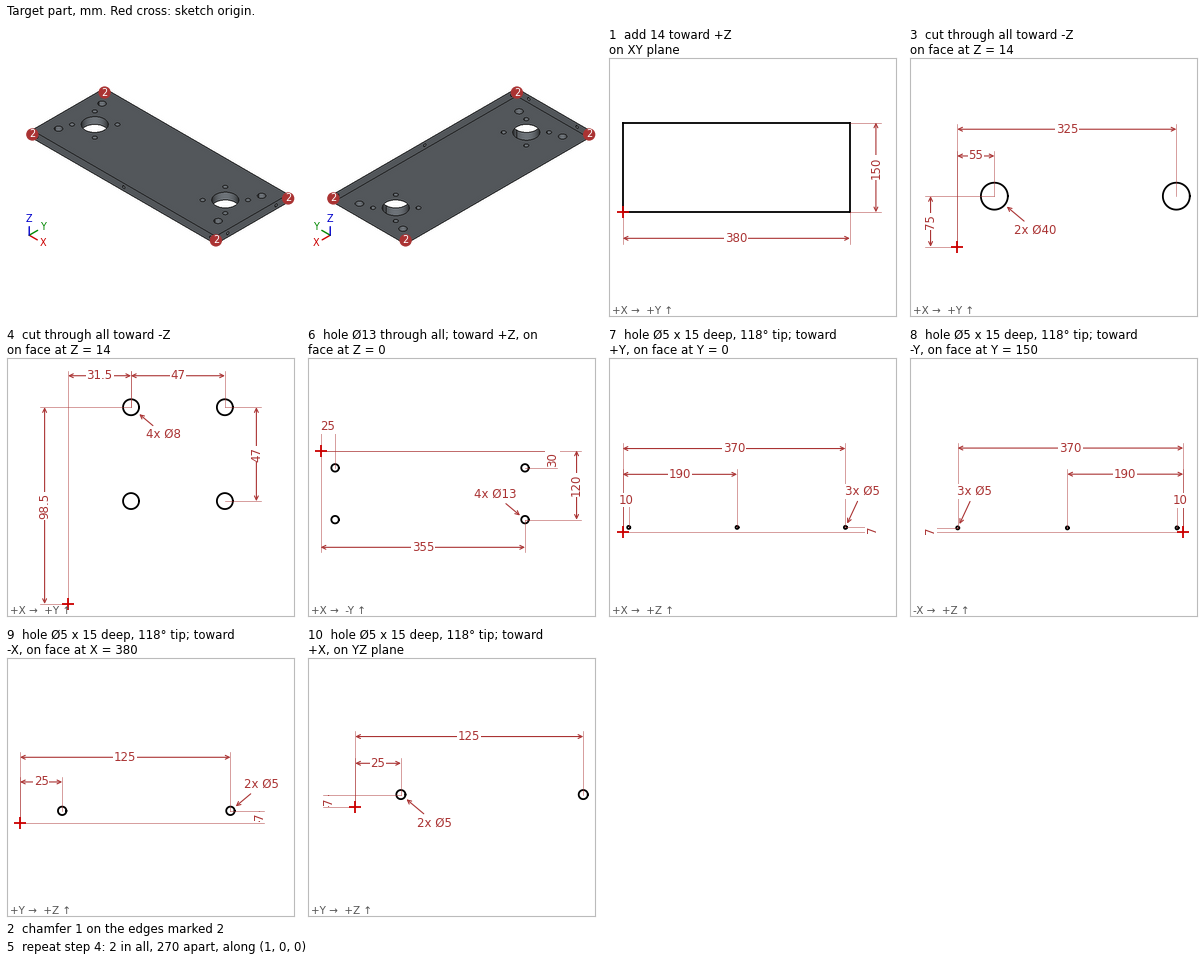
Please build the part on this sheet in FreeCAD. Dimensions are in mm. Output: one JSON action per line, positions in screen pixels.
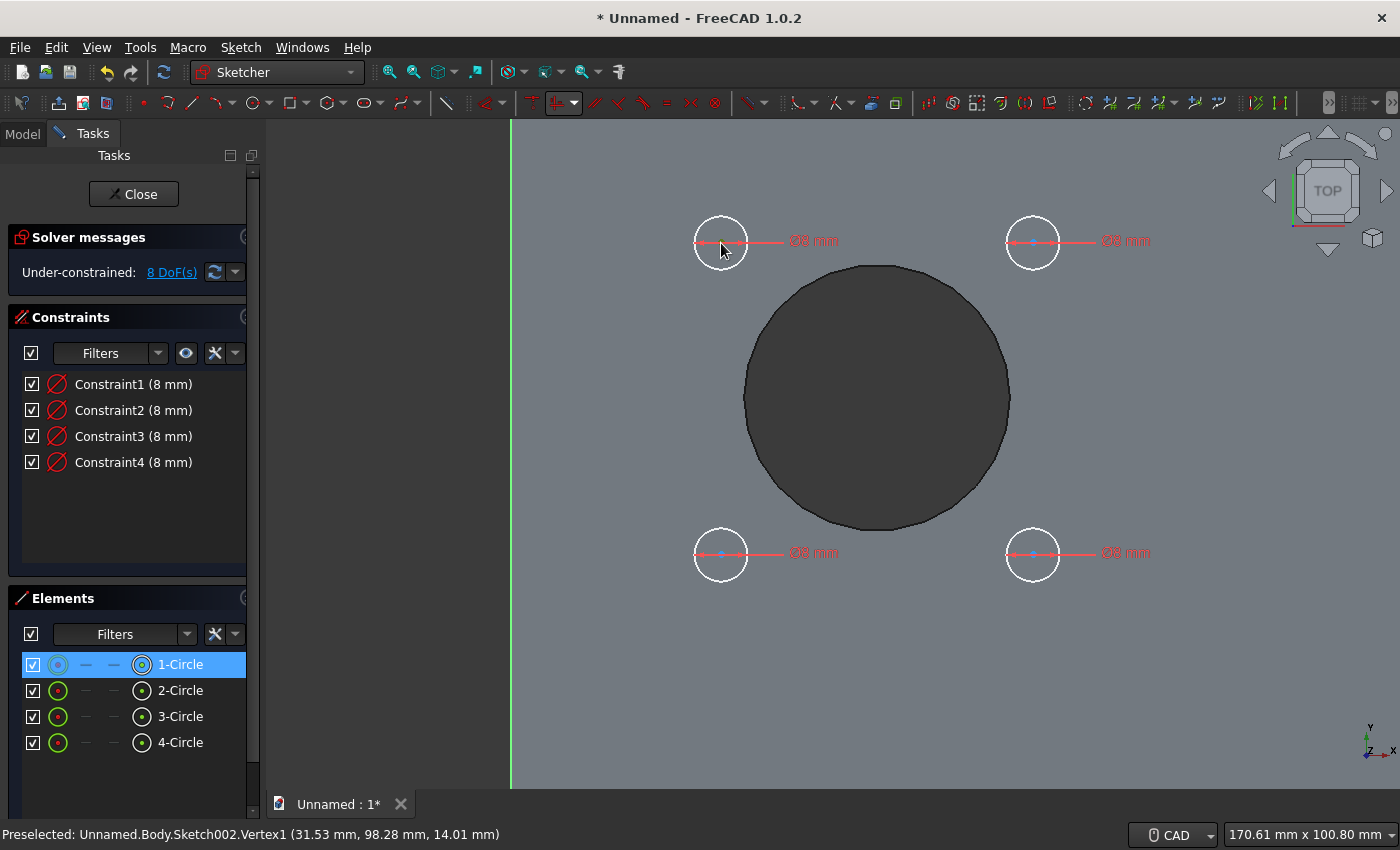
{"action": "left_click", "coordinate": [1033, 243]}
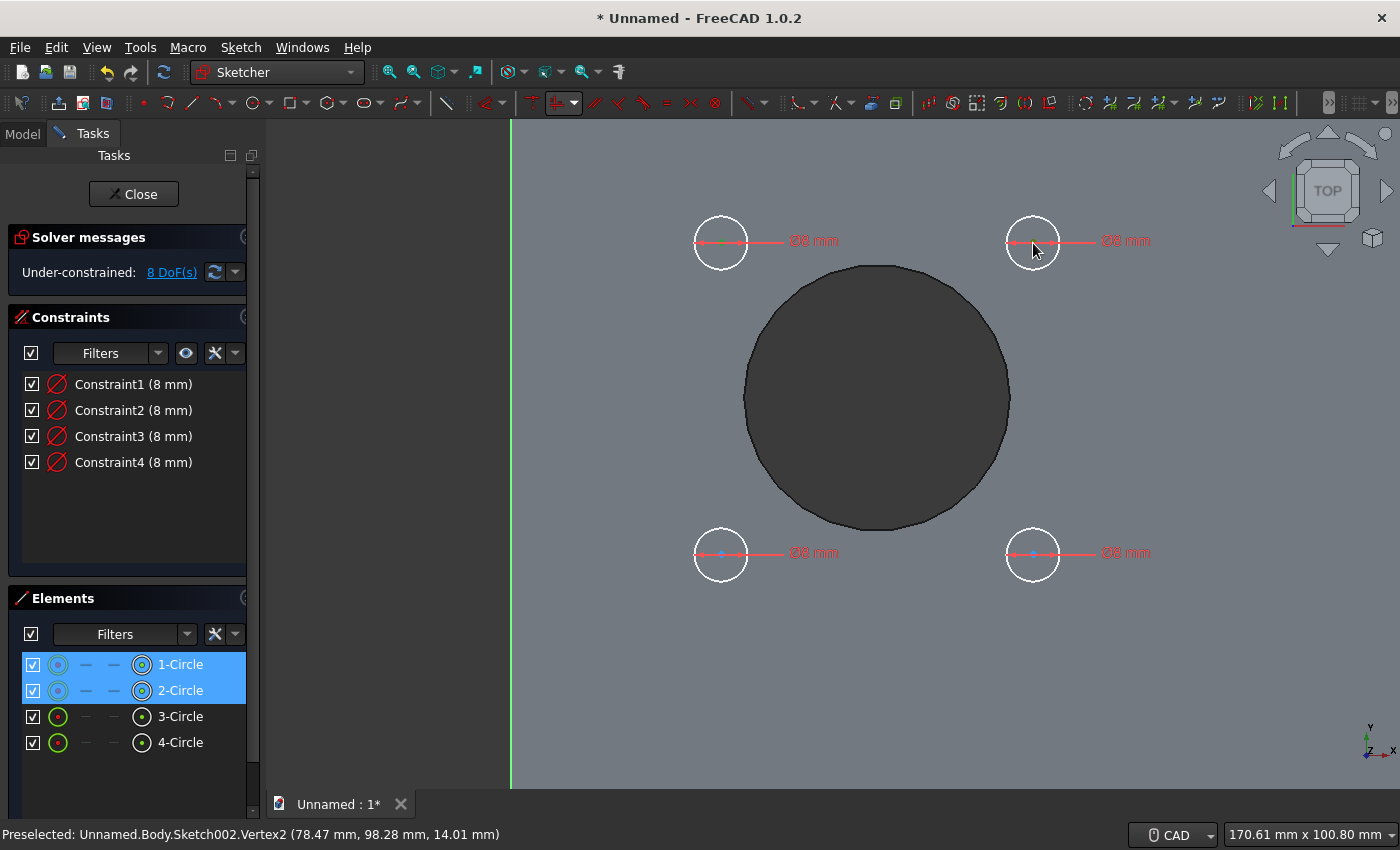
{"action": "left_click", "coordinate": [576, 104]}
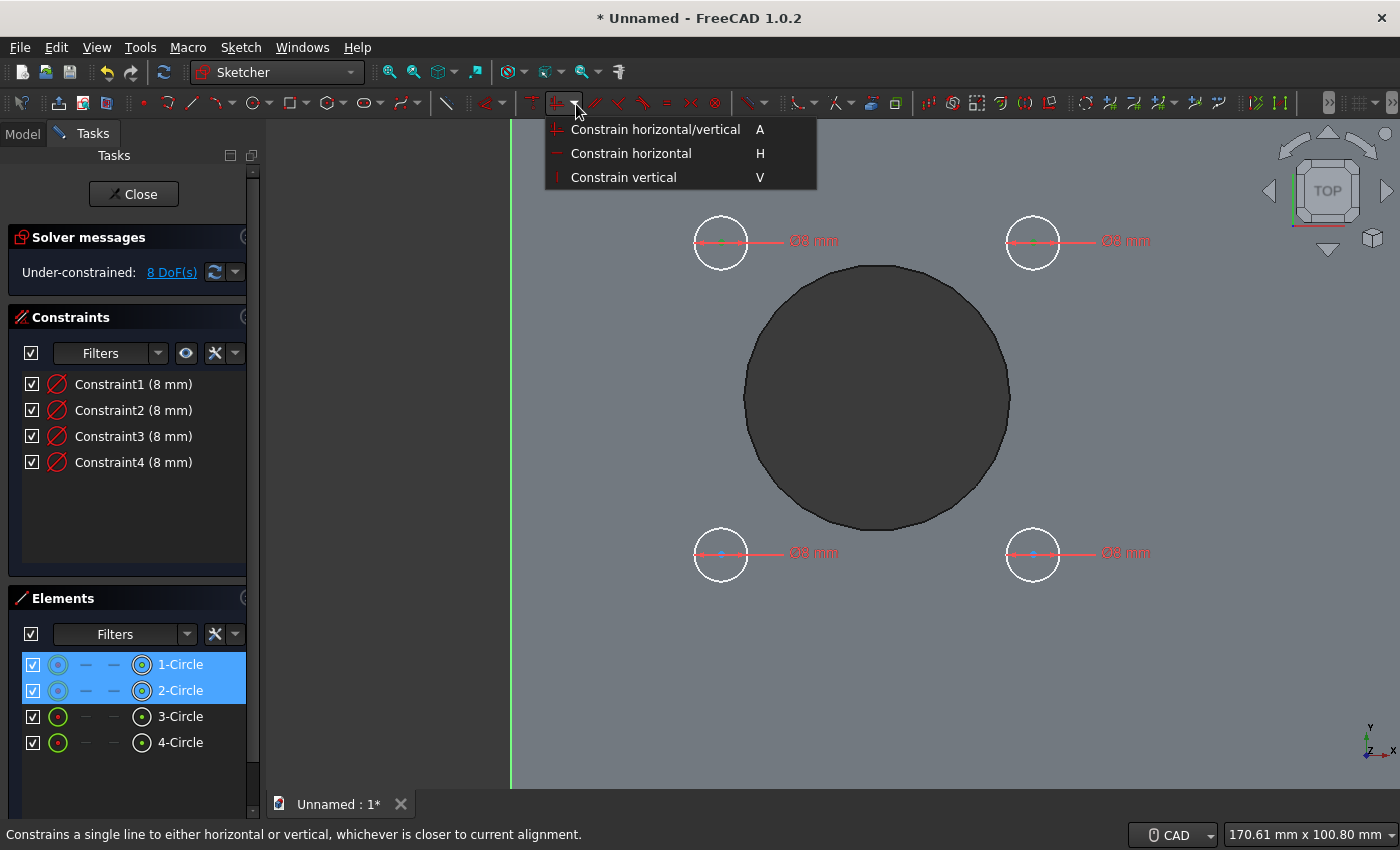
{"action": "left_click", "coordinate": [681, 153]}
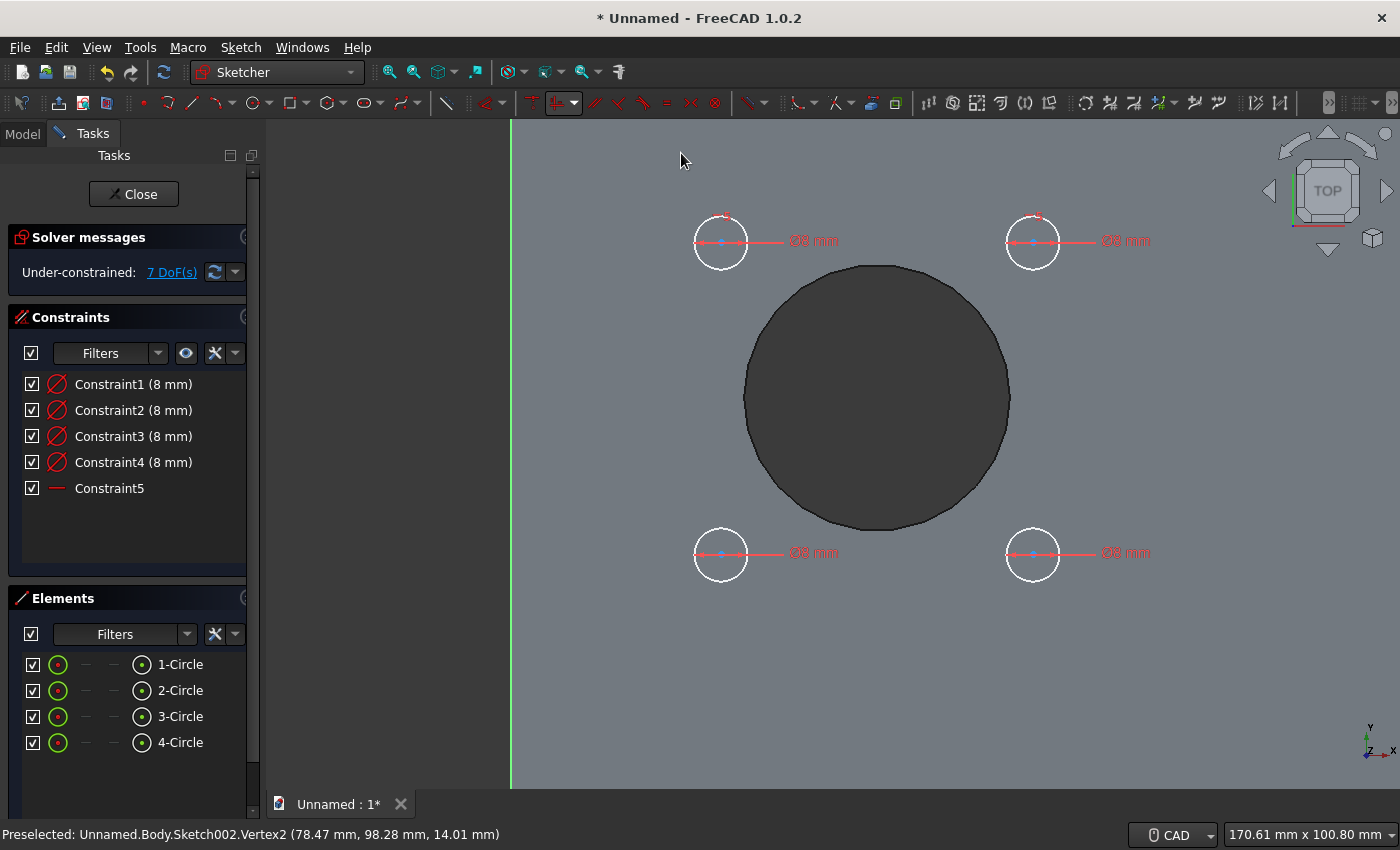
{"action": "left_click", "coordinate": [1033, 243]}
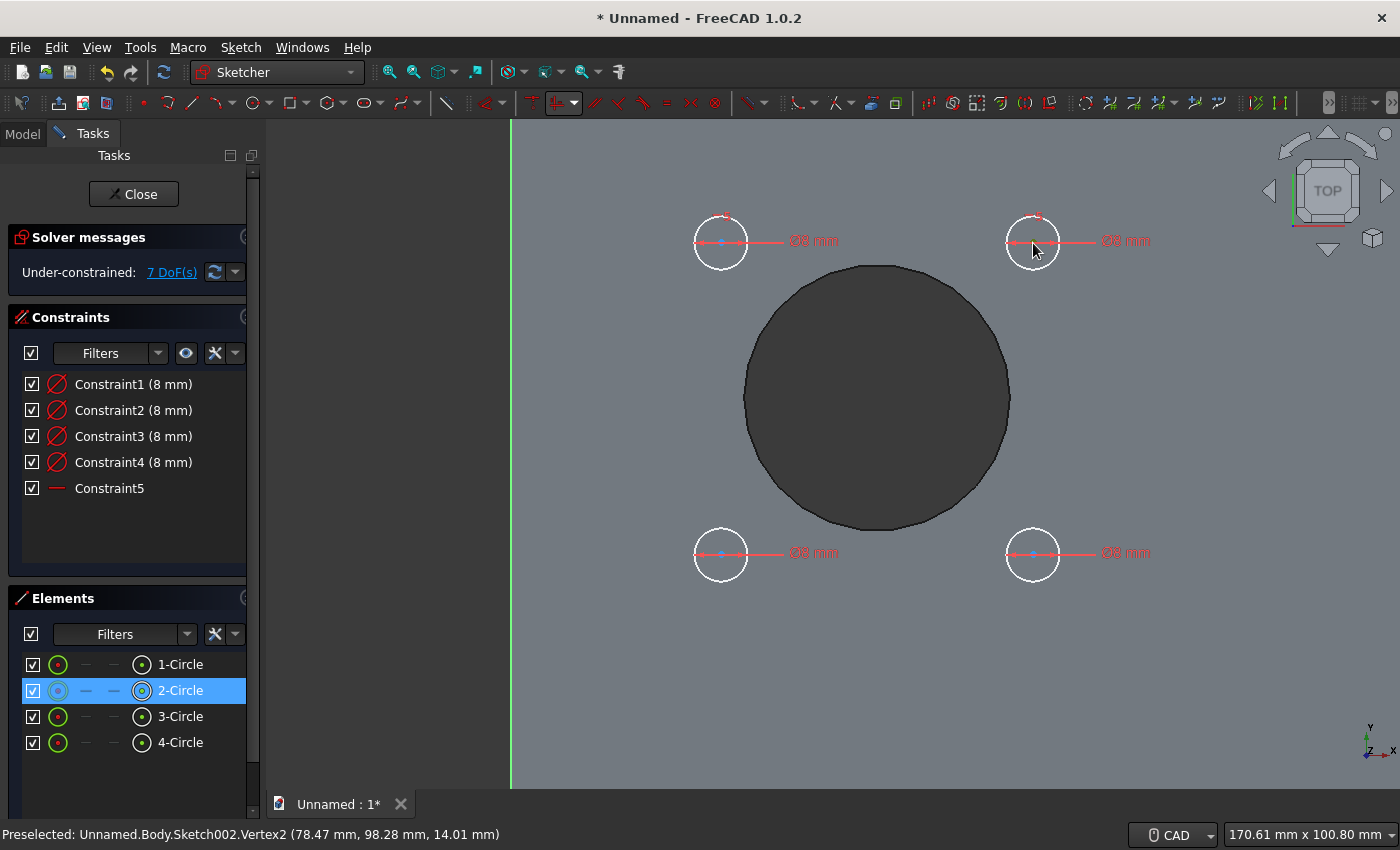
{"action": "left_click", "coordinate": [1033, 555]}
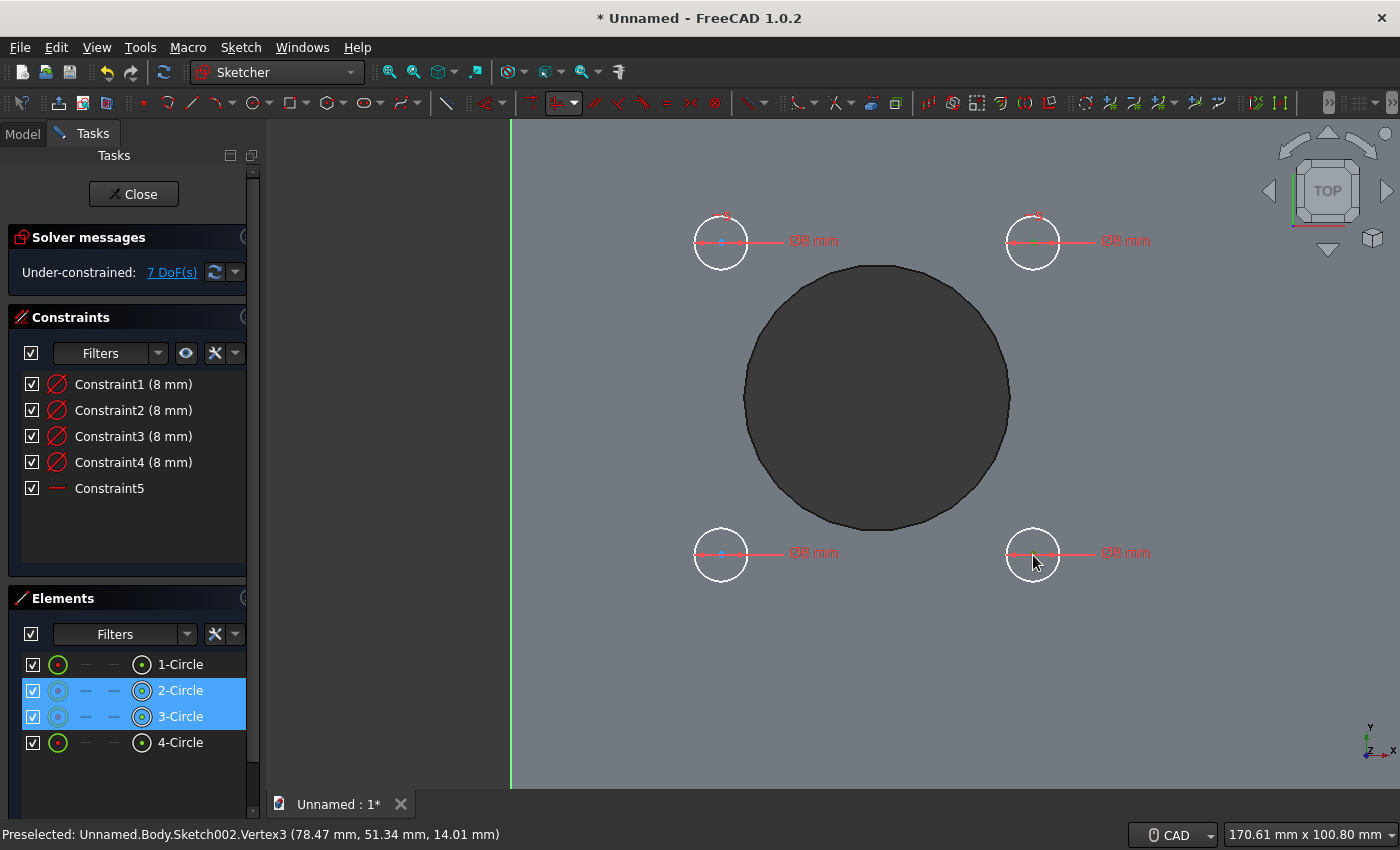
{"action": "key", "text": "v"}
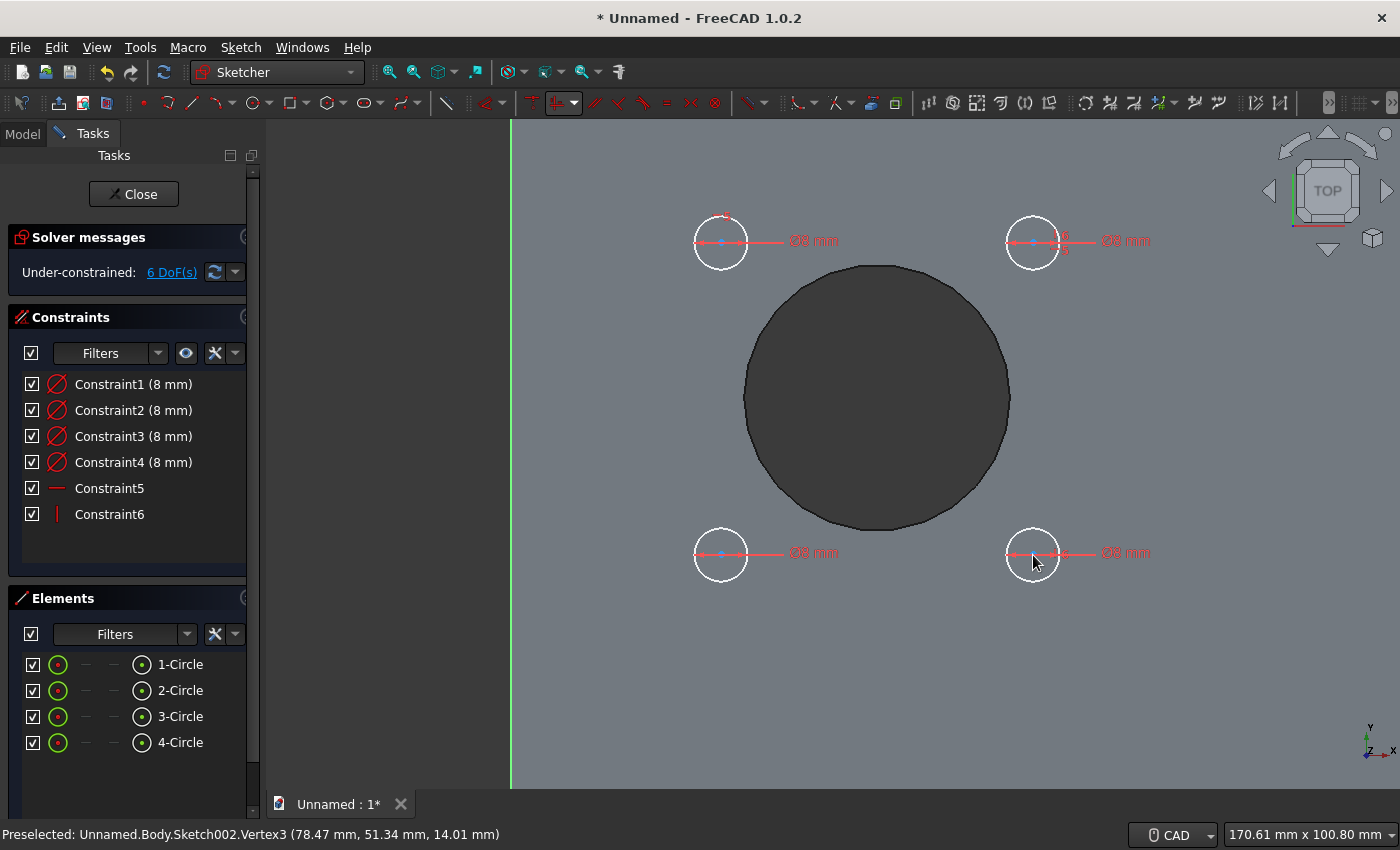
{"action": "left_click", "coordinate": [721, 243]}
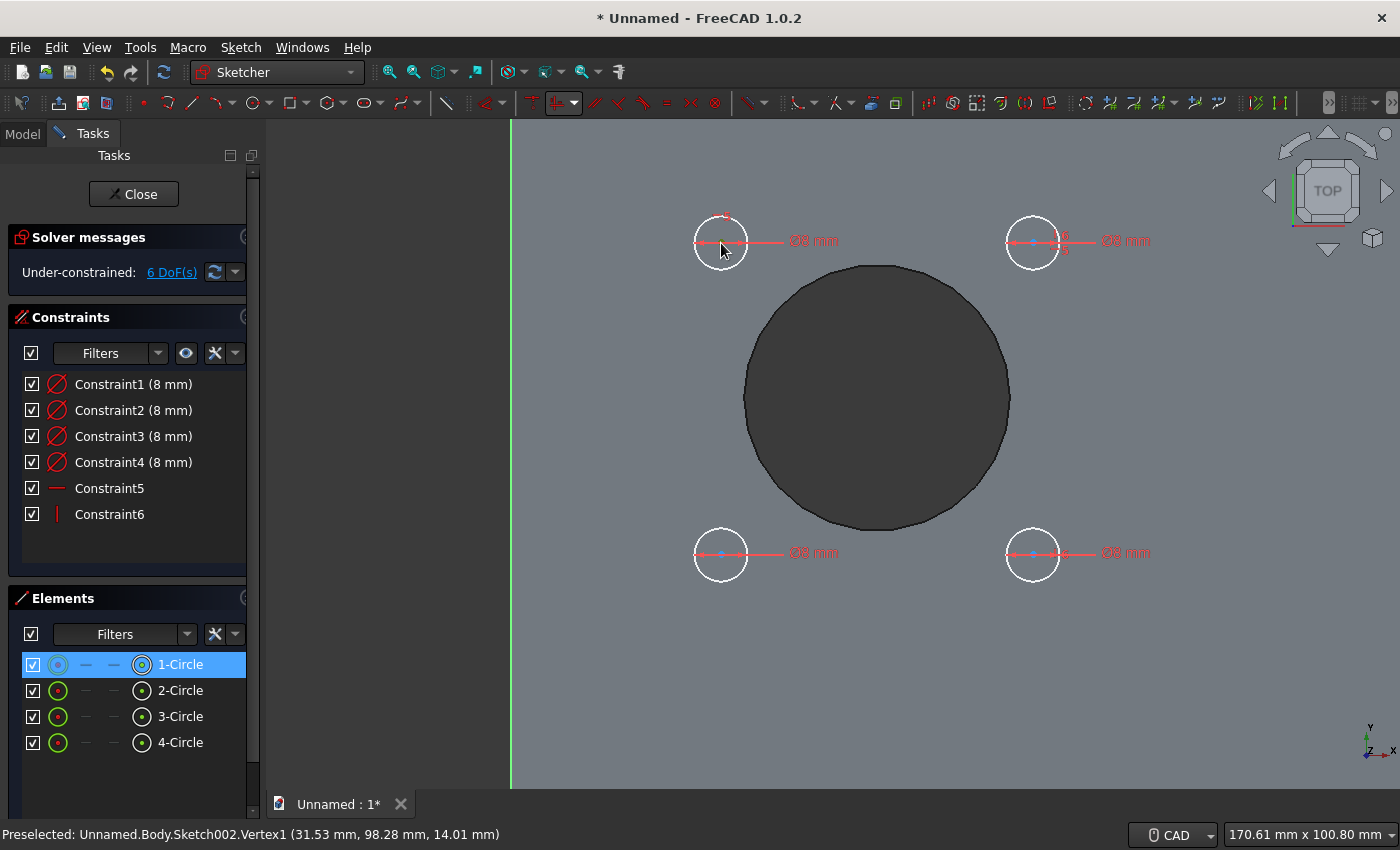
{"action": "left_click", "coordinate": [721, 555]}